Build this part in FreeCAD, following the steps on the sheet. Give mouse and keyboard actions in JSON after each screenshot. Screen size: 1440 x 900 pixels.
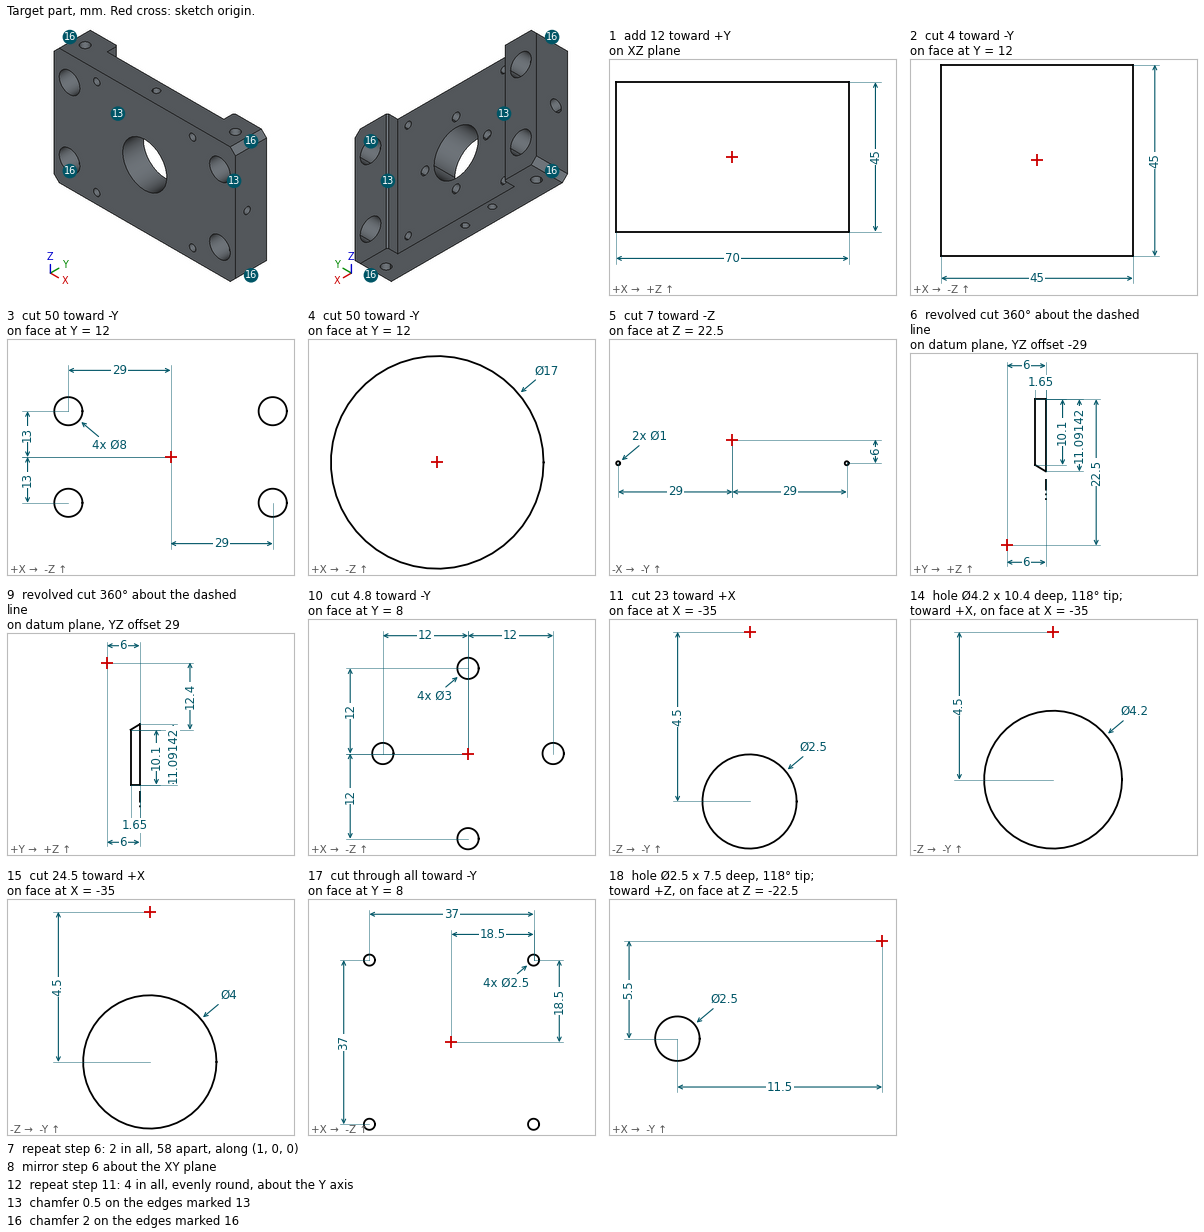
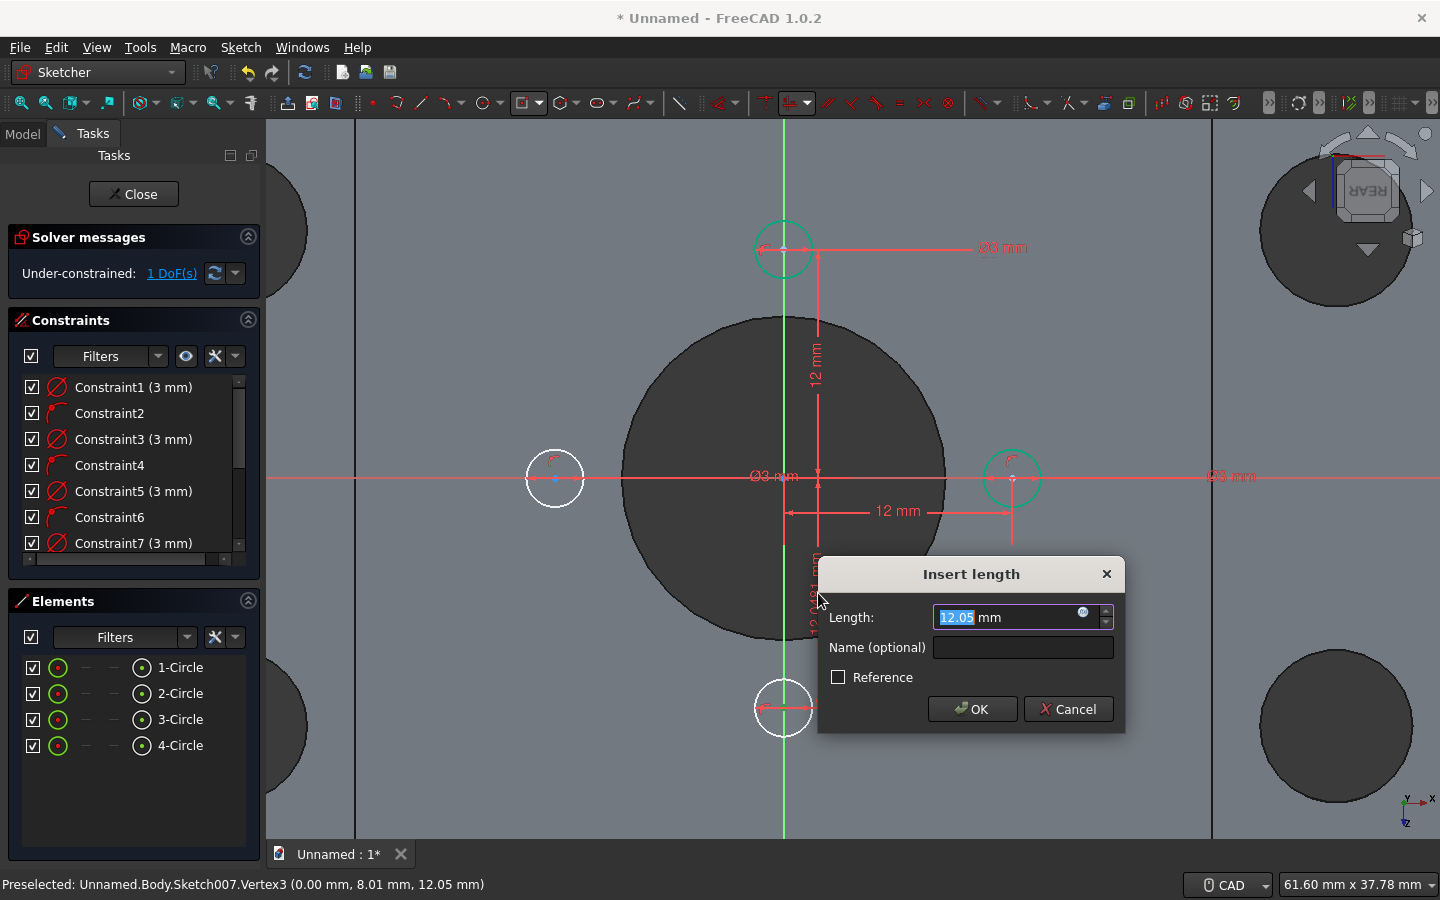
{"action": "type", "text": "12"}
{"action": "key", "text": "Return"}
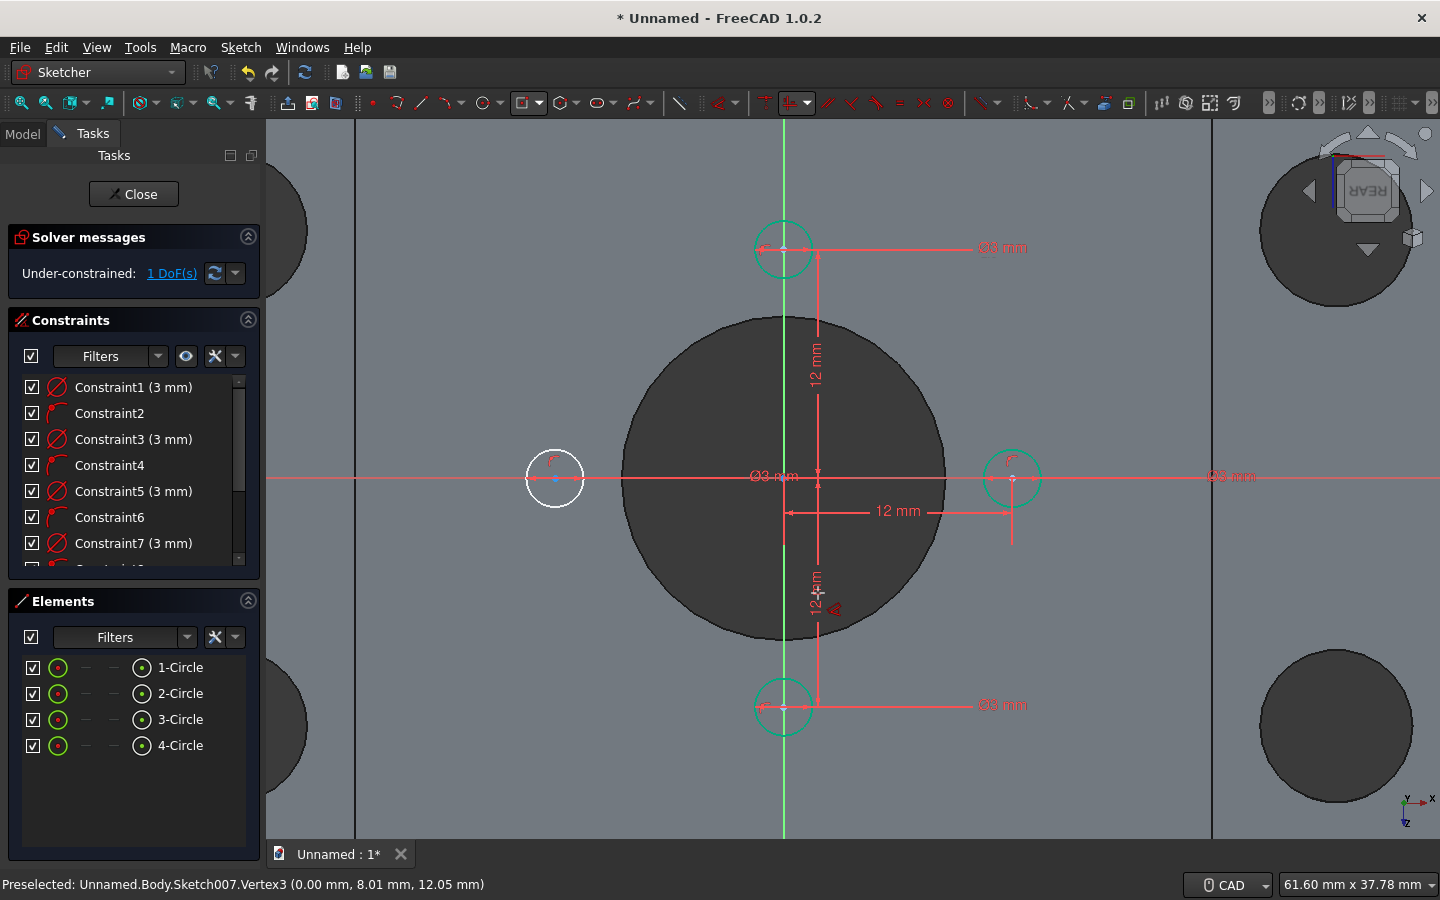
{"action": "left_click", "coordinate": [555, 478]}
{"action": "left_click", "coordinate": [669, 512]}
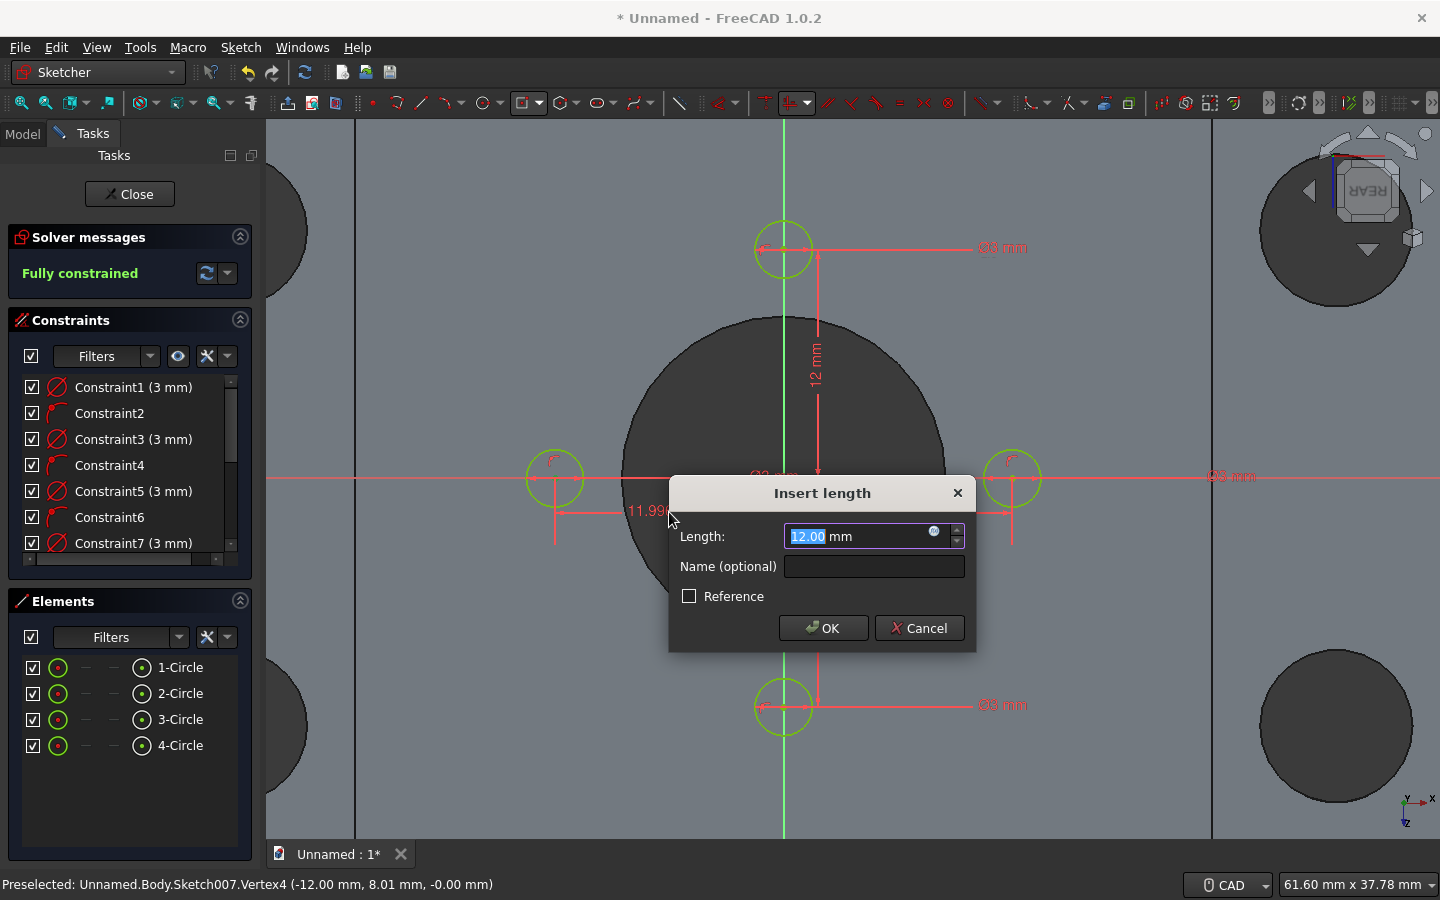
{"action": "type", "text": "12"}
{"action": "key", "text": "Return"}
{"action": "key", "text": "Escape"}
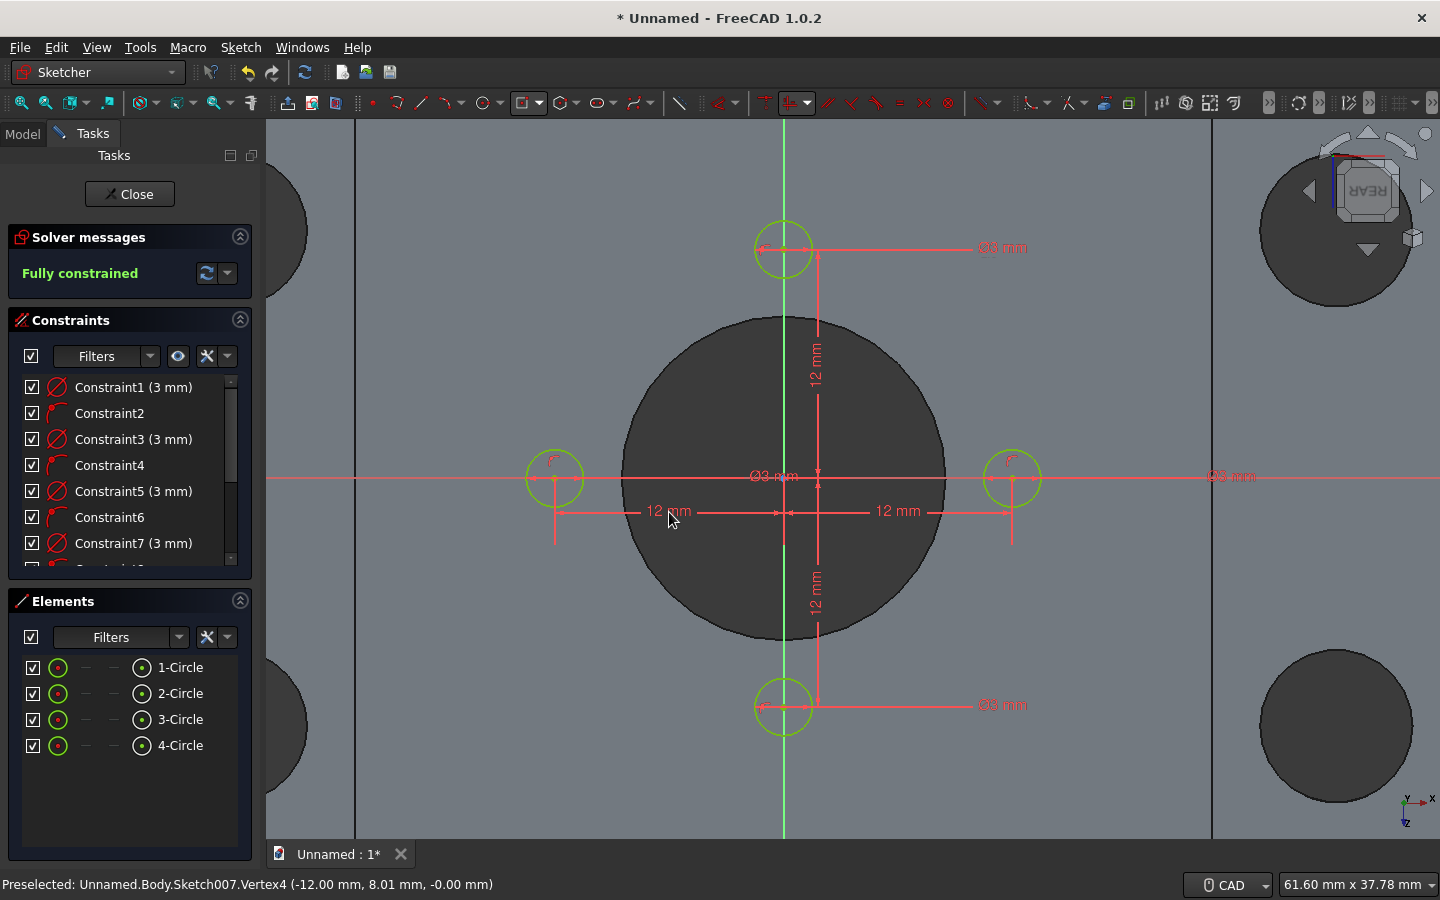
{"action": "left_click", "coordinate": [130, 194]}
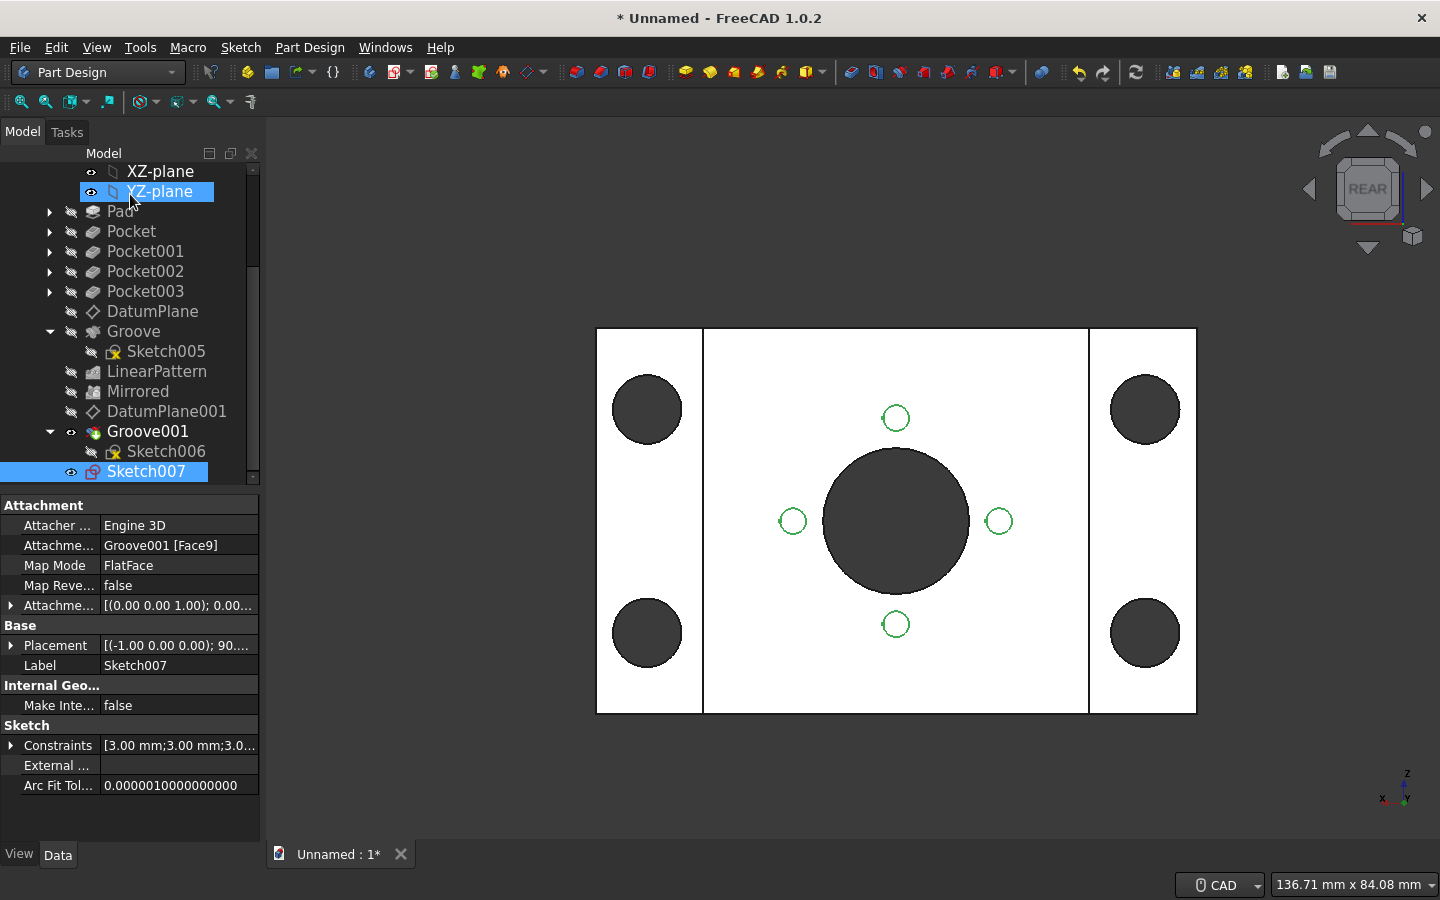
{"action": "left_click", "coordinate": [852, 72]}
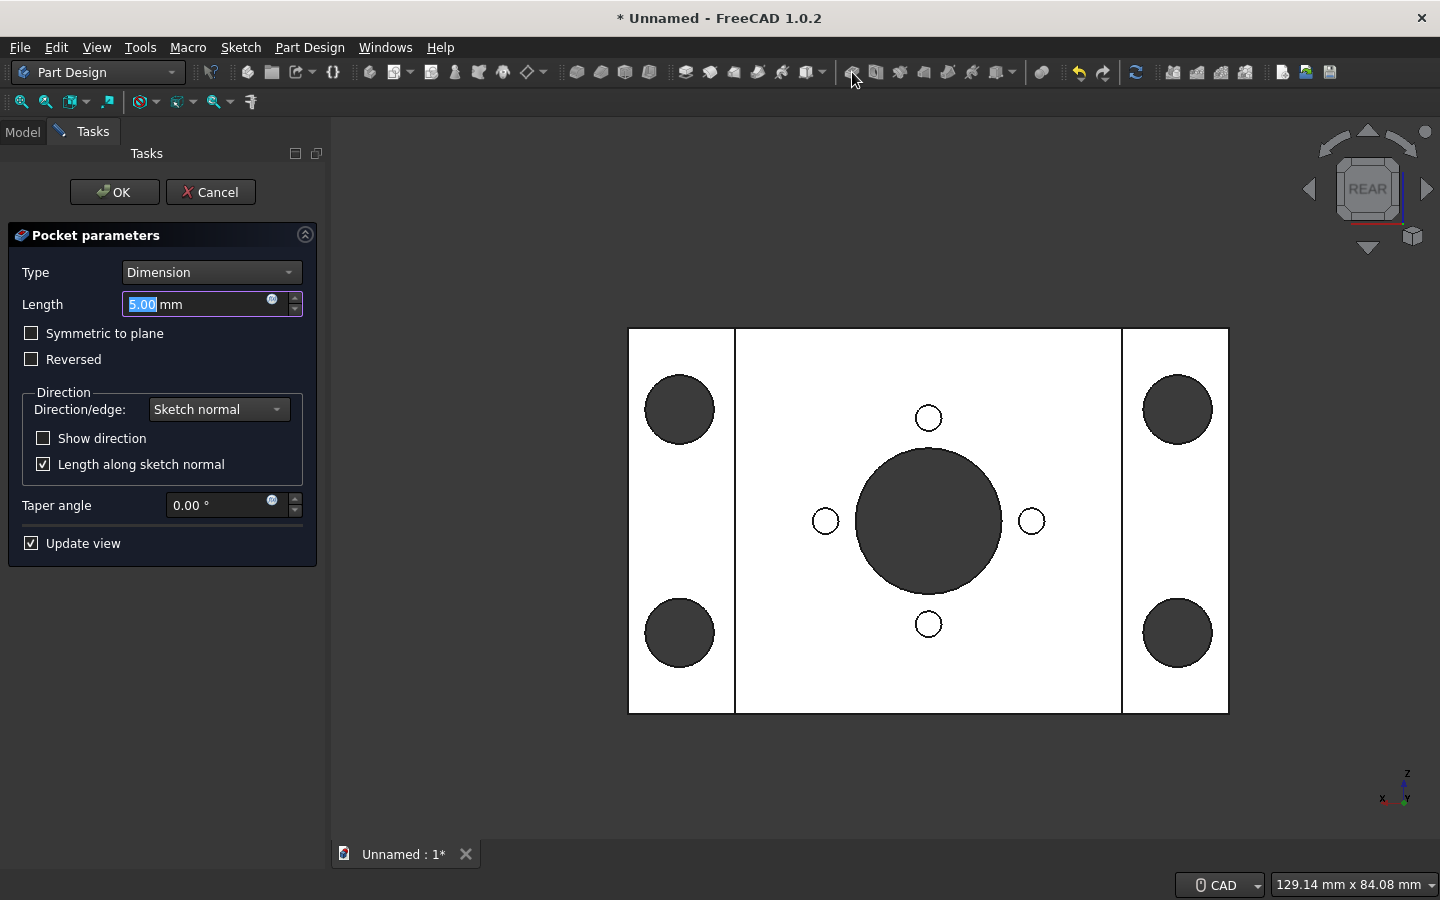
{"action": "type", "text": "4.8"}
{"action": "key", "text": "Tab"}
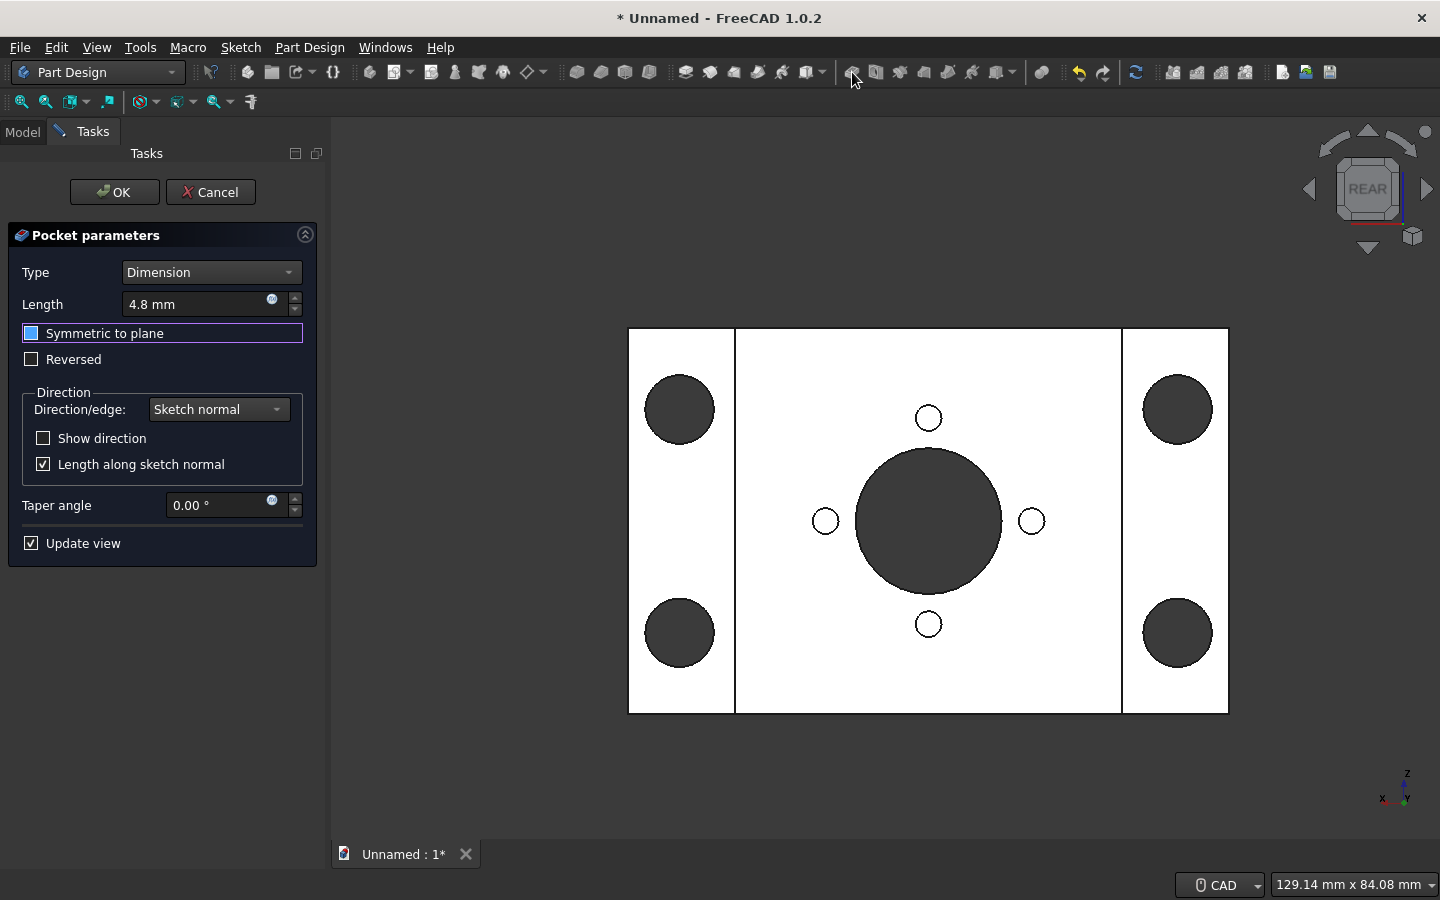
{"action": "left_click", "coordinate": [115, 192]}